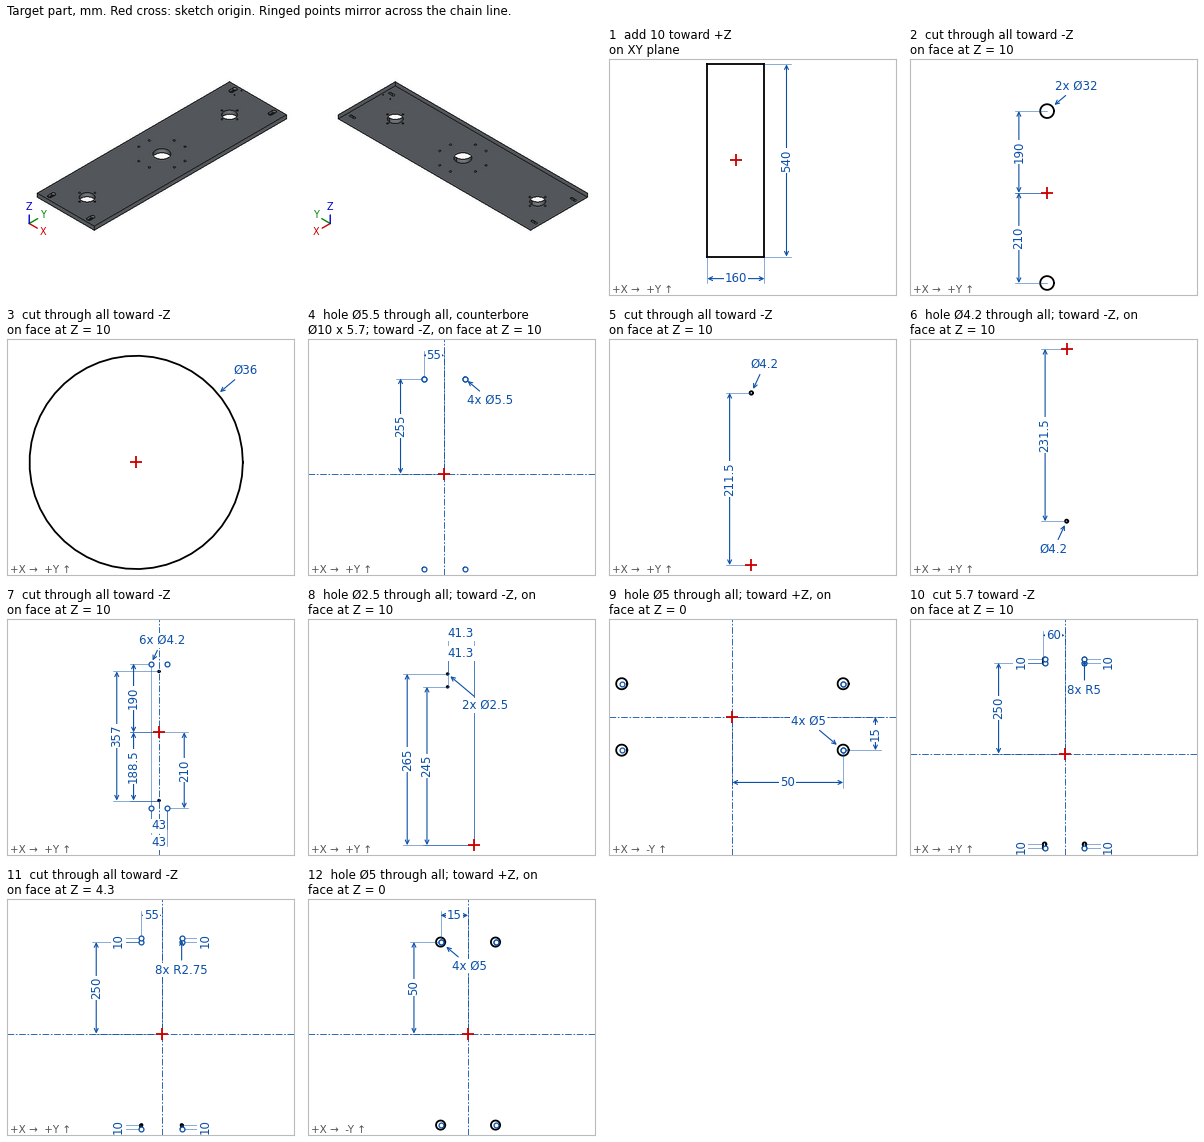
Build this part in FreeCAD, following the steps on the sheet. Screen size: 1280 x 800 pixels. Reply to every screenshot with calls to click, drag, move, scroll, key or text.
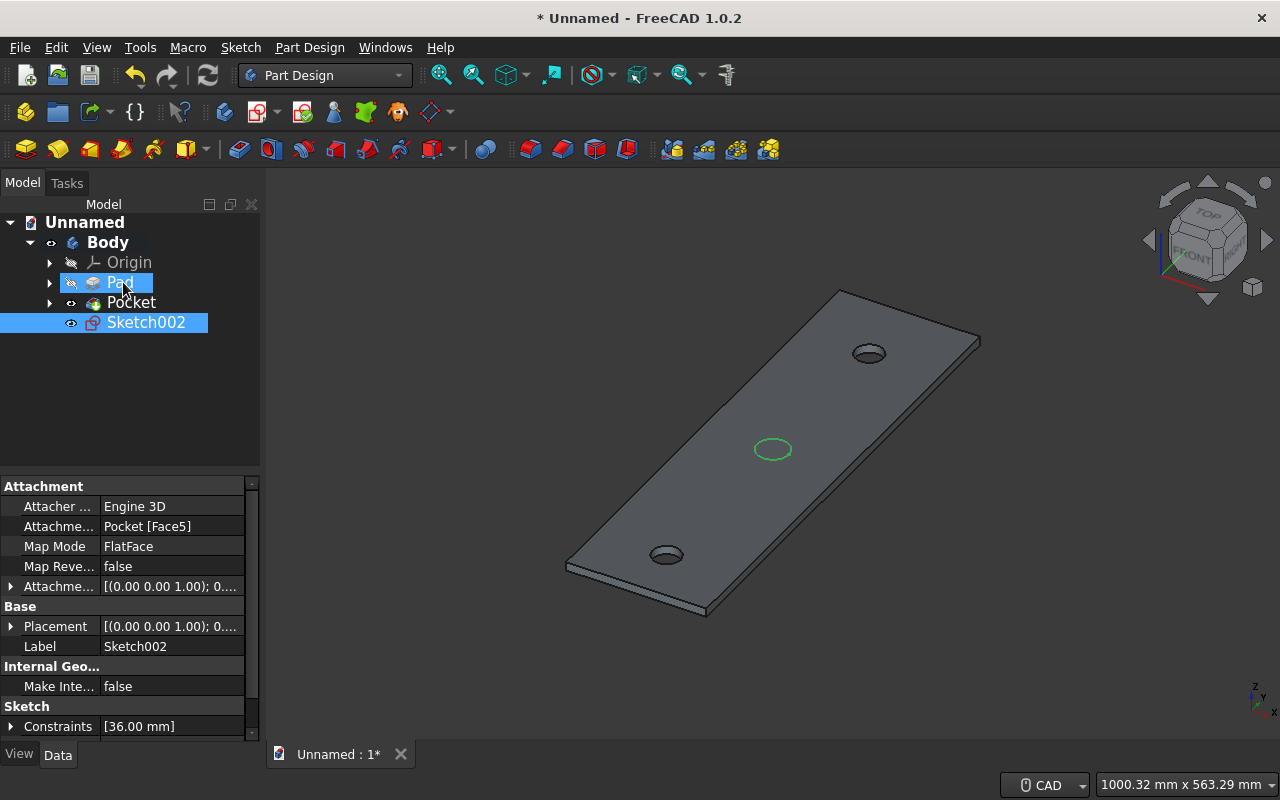
click(240, 150)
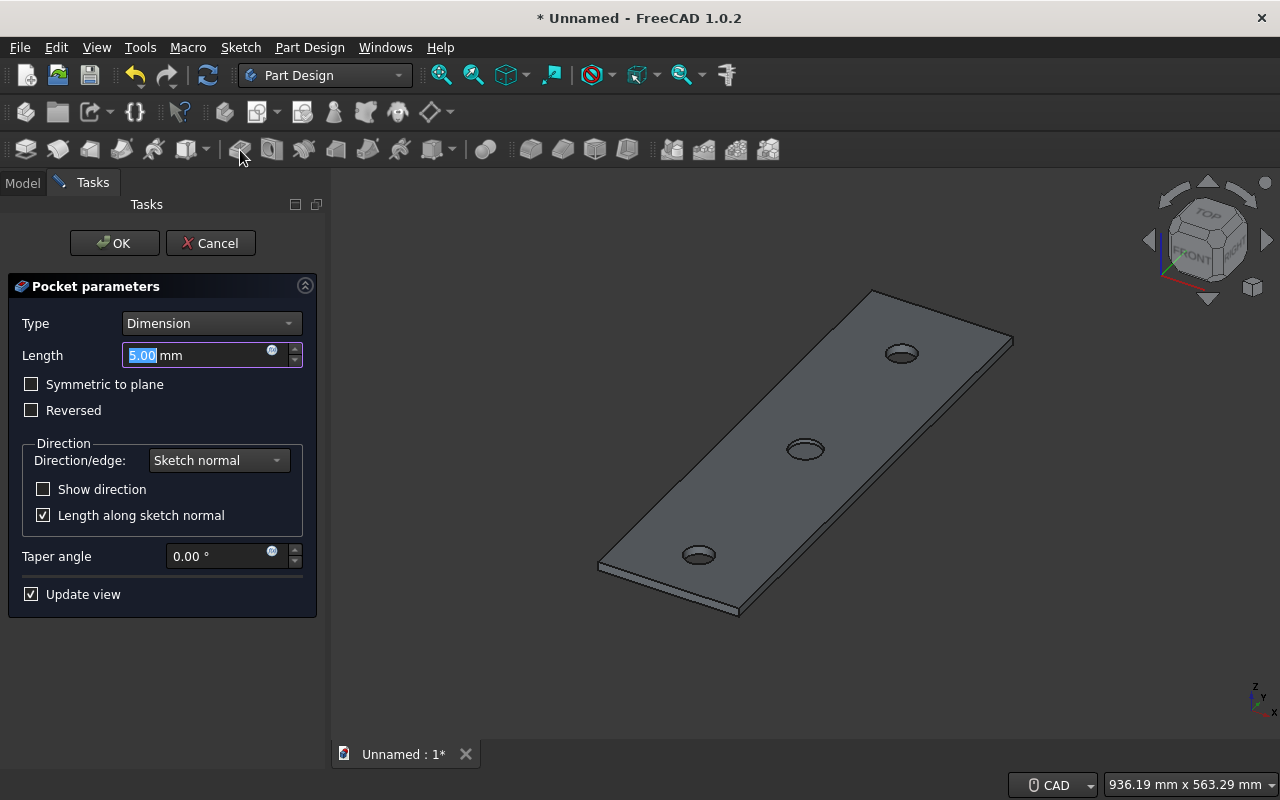
click(212, 324)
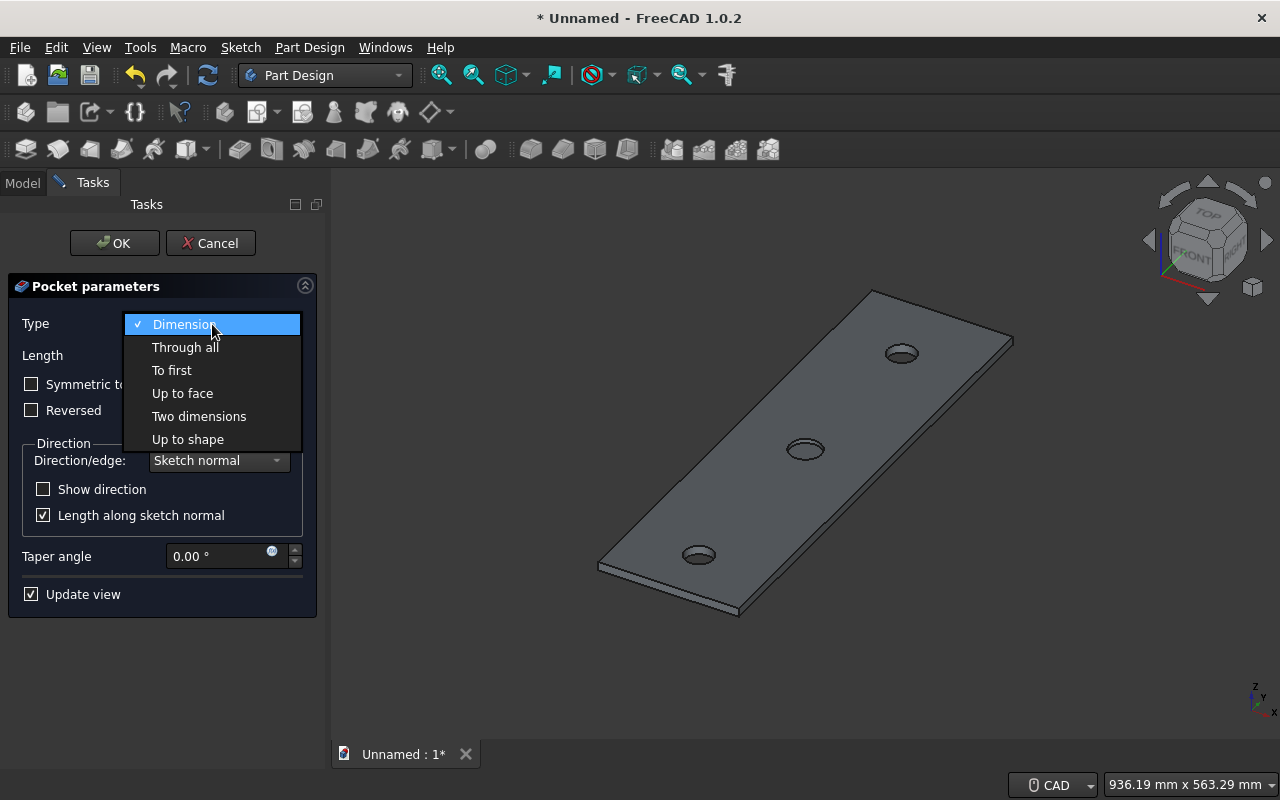
click(212, 348)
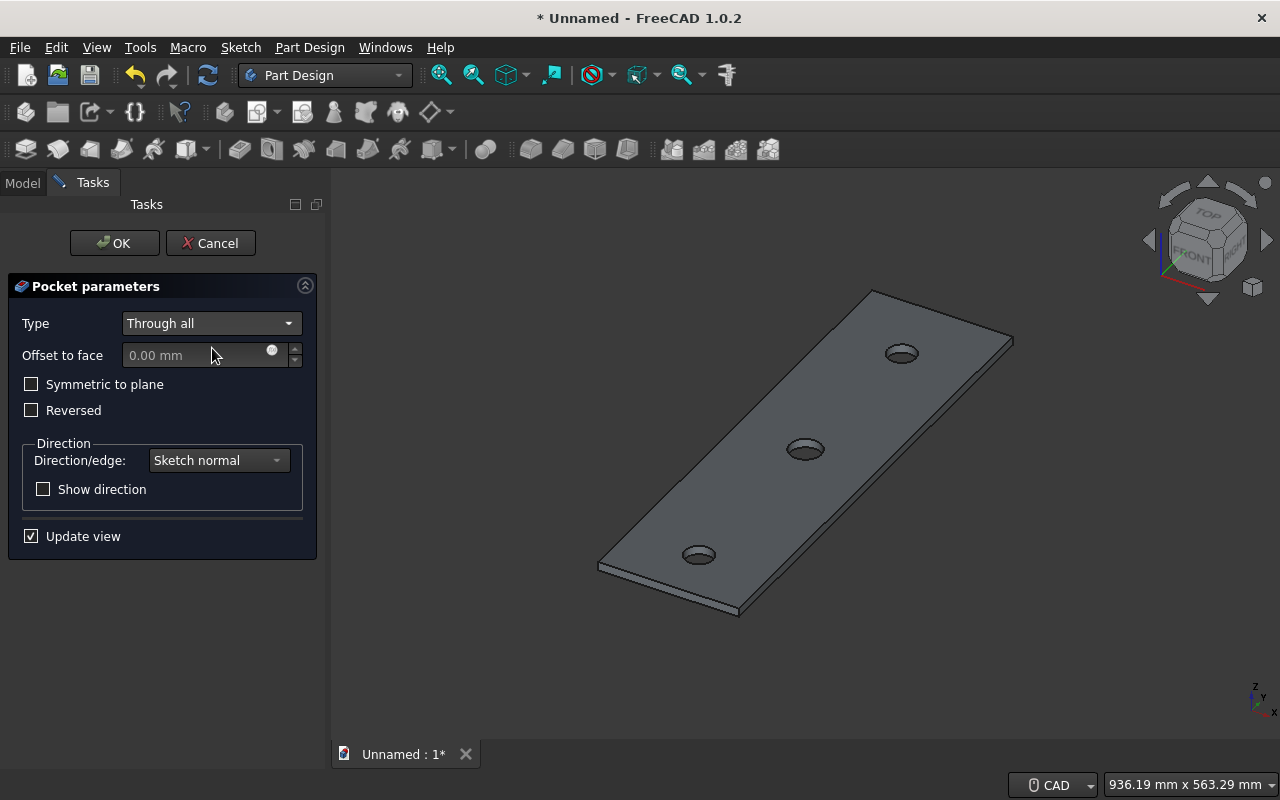
click(115, 243)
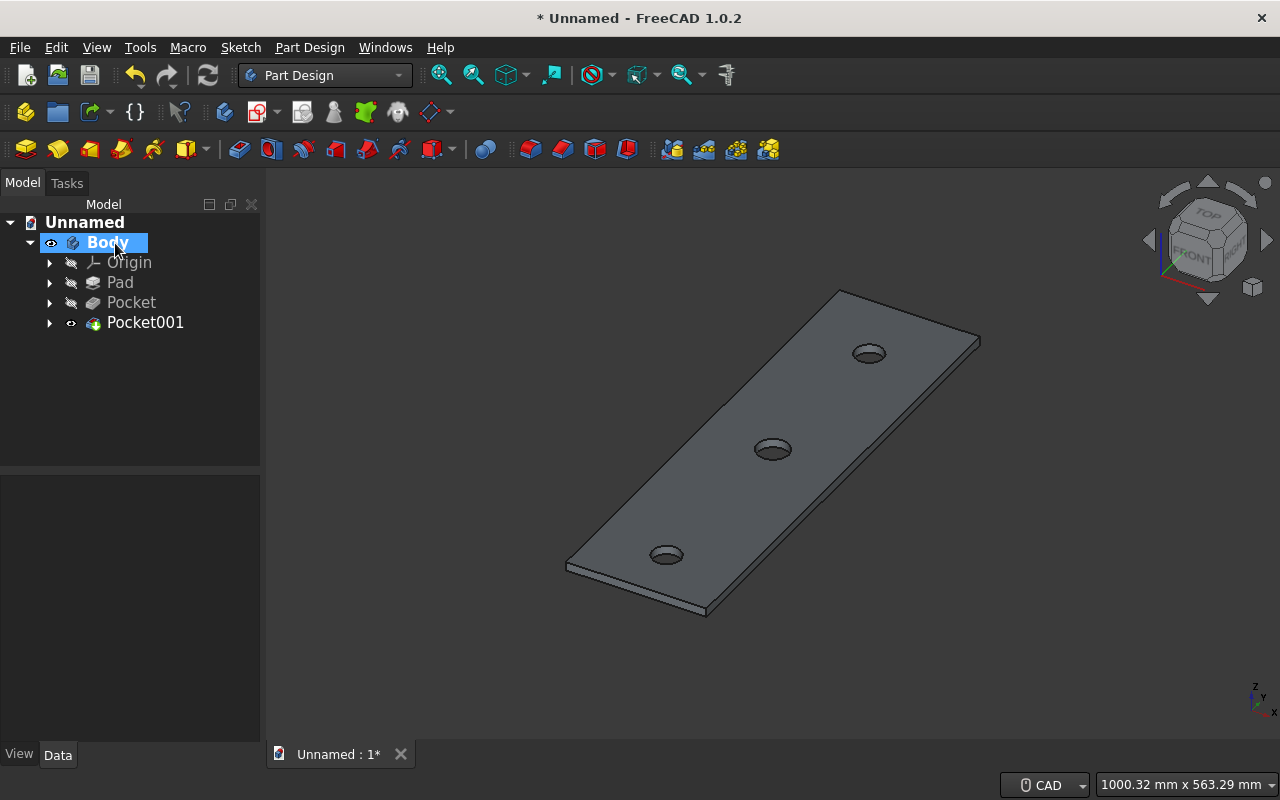
click(812, 410)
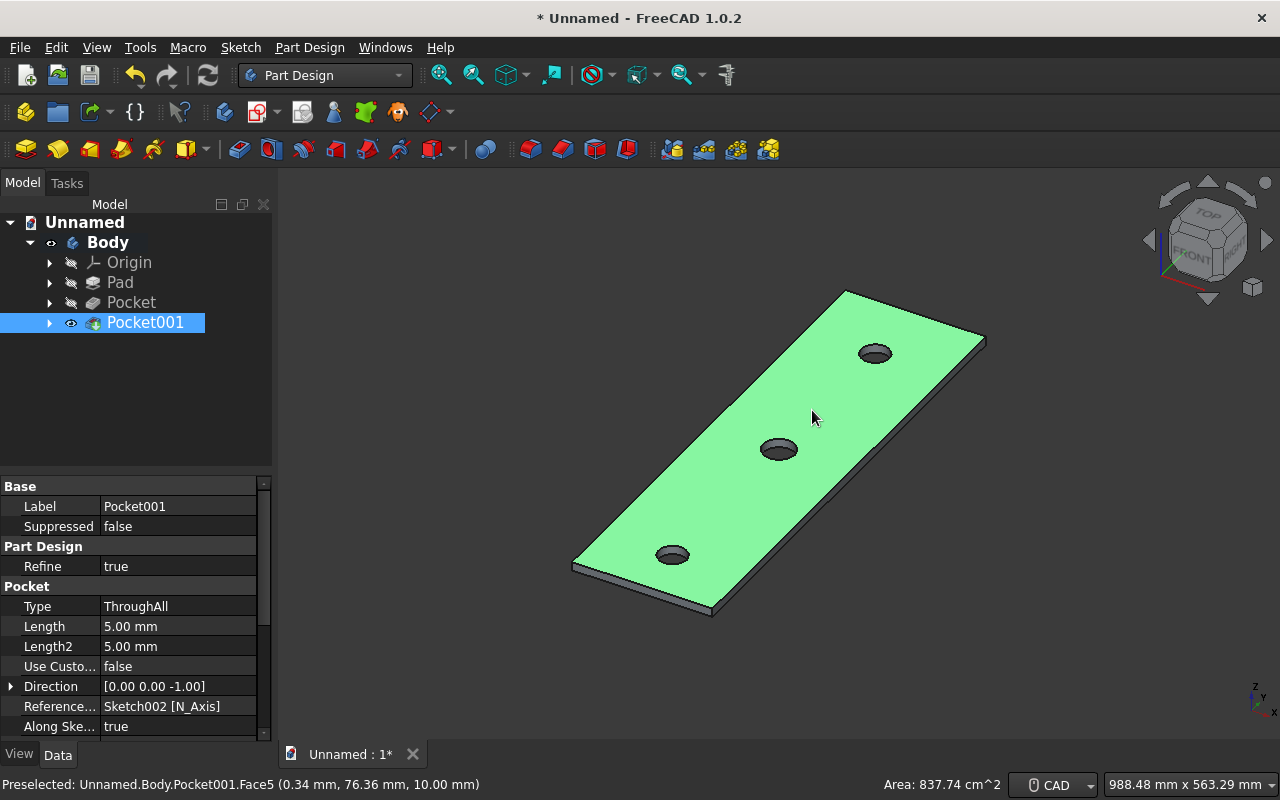
click(258, 112)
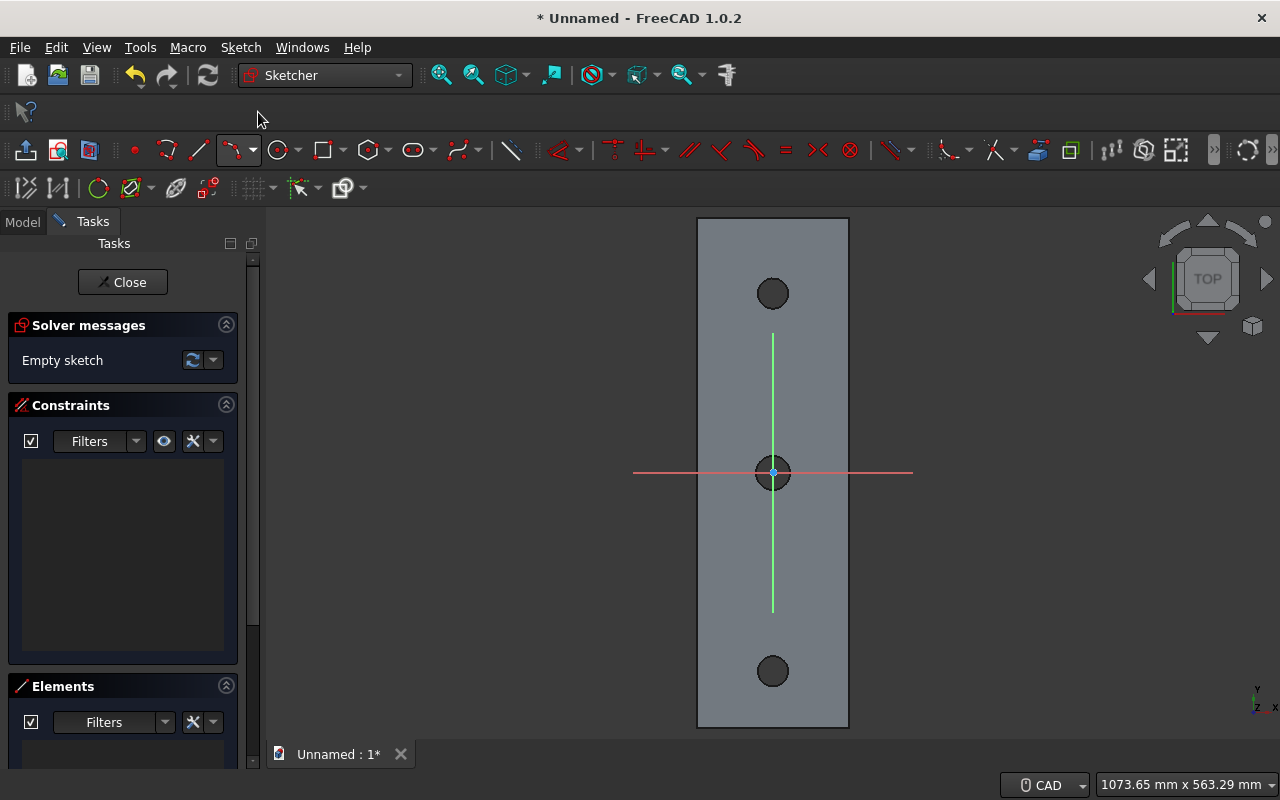
scroll(565, 473, down, 2)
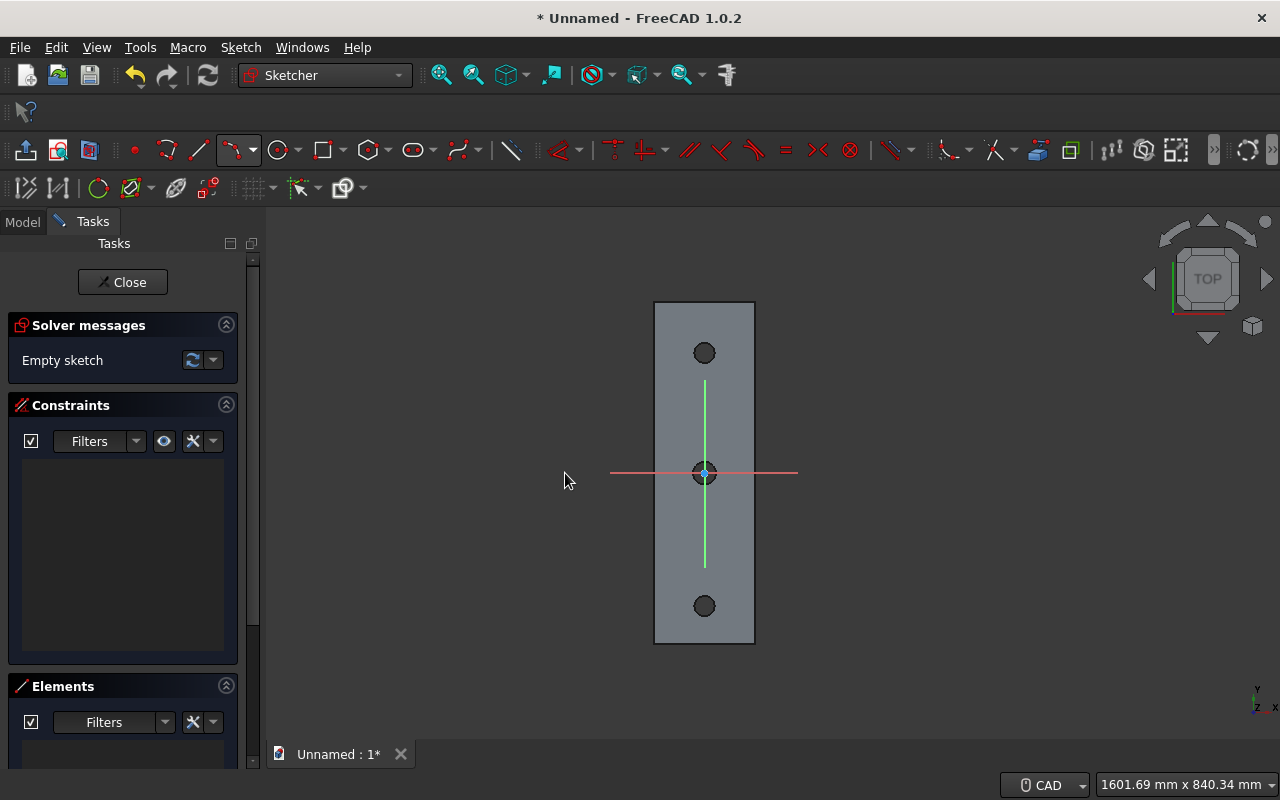
key(g)
key(c)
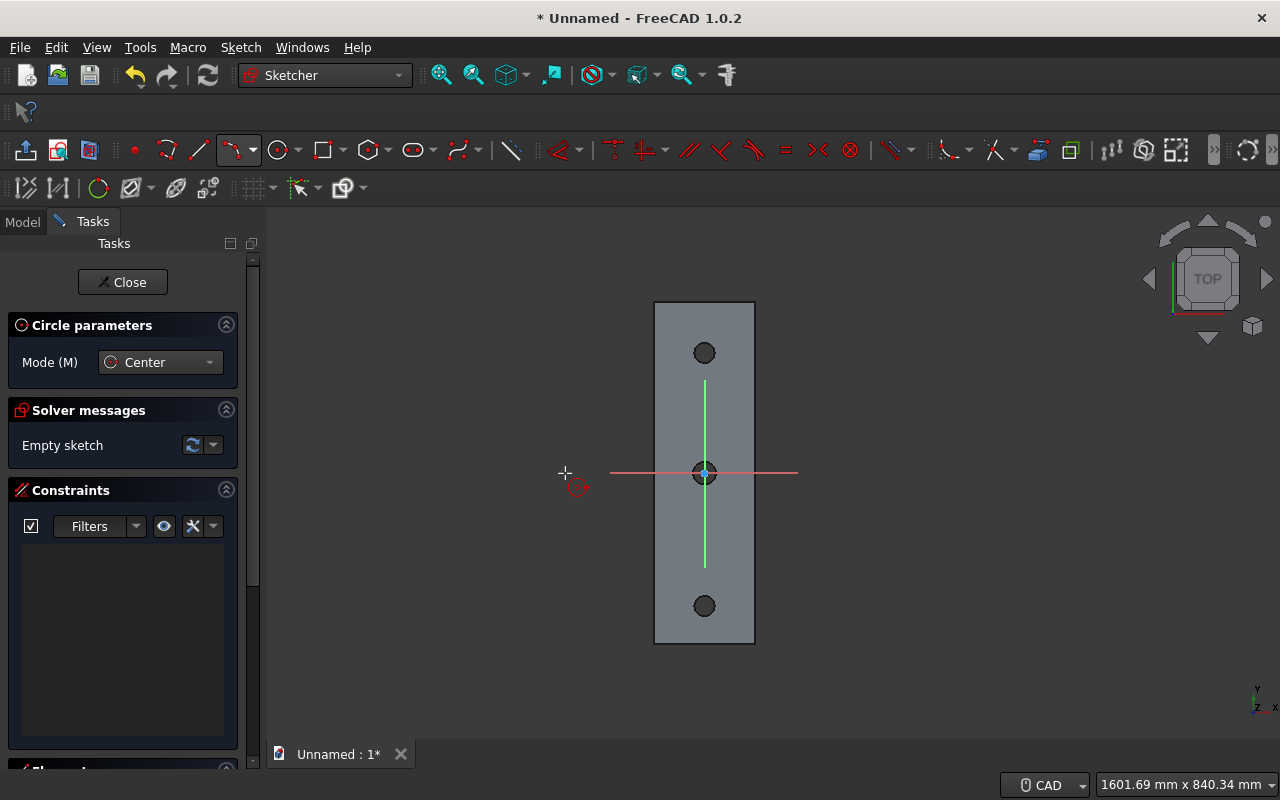
scroll(670, 312, up, 13)